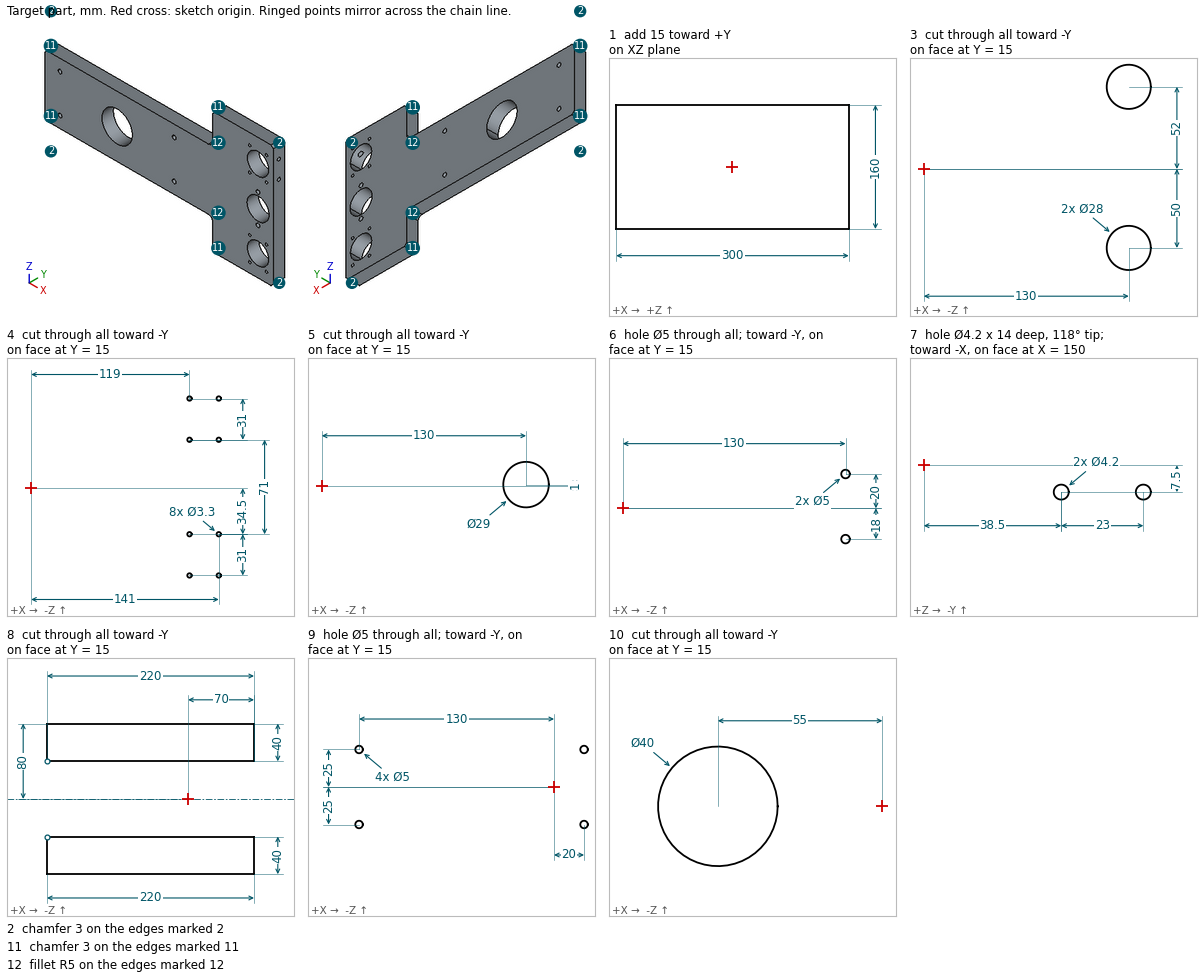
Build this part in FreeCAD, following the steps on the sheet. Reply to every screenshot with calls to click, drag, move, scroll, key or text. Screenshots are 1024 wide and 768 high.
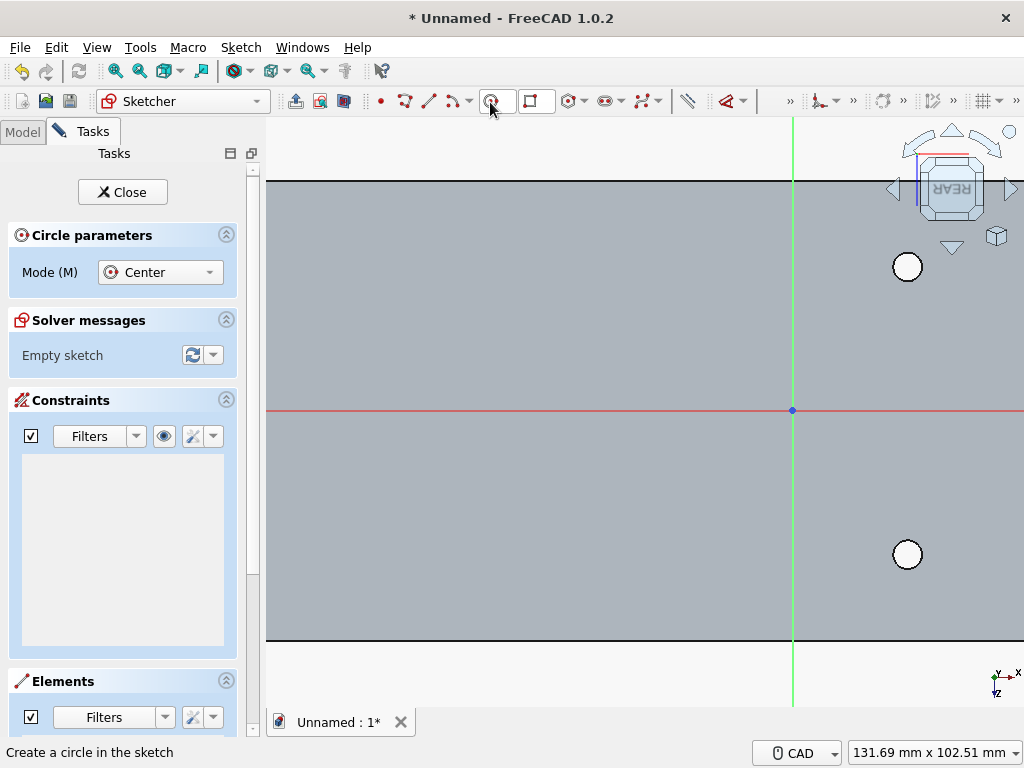
click(476, 411)
move(557, 329)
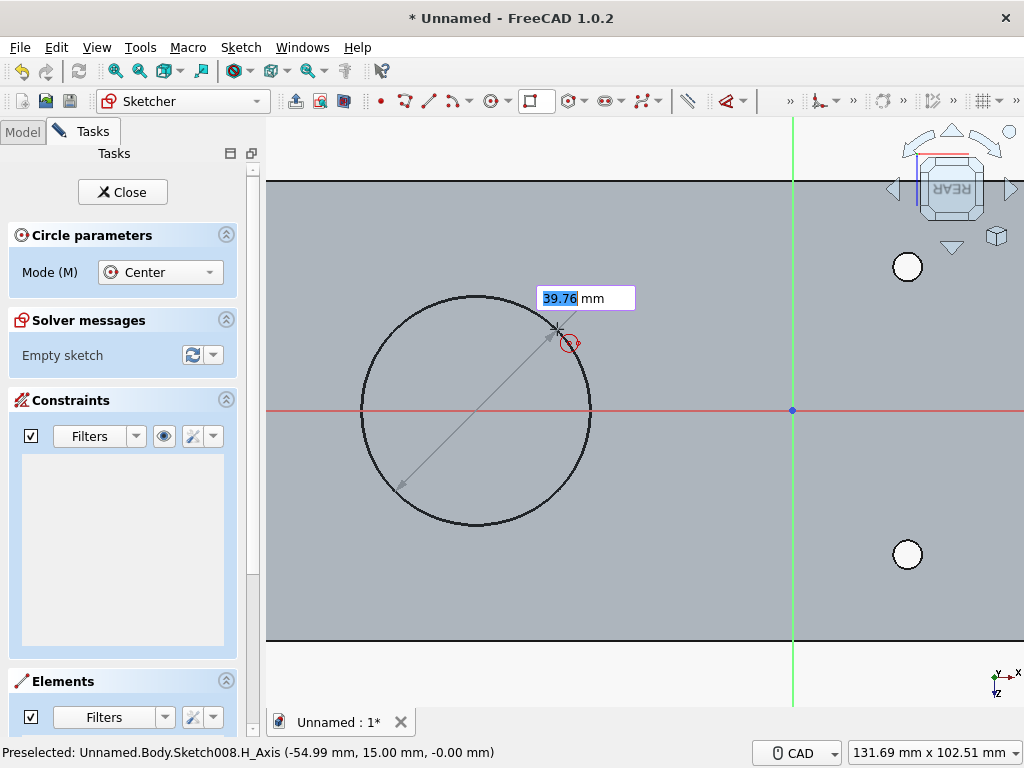
text(40)
key(Return)
key(Escape)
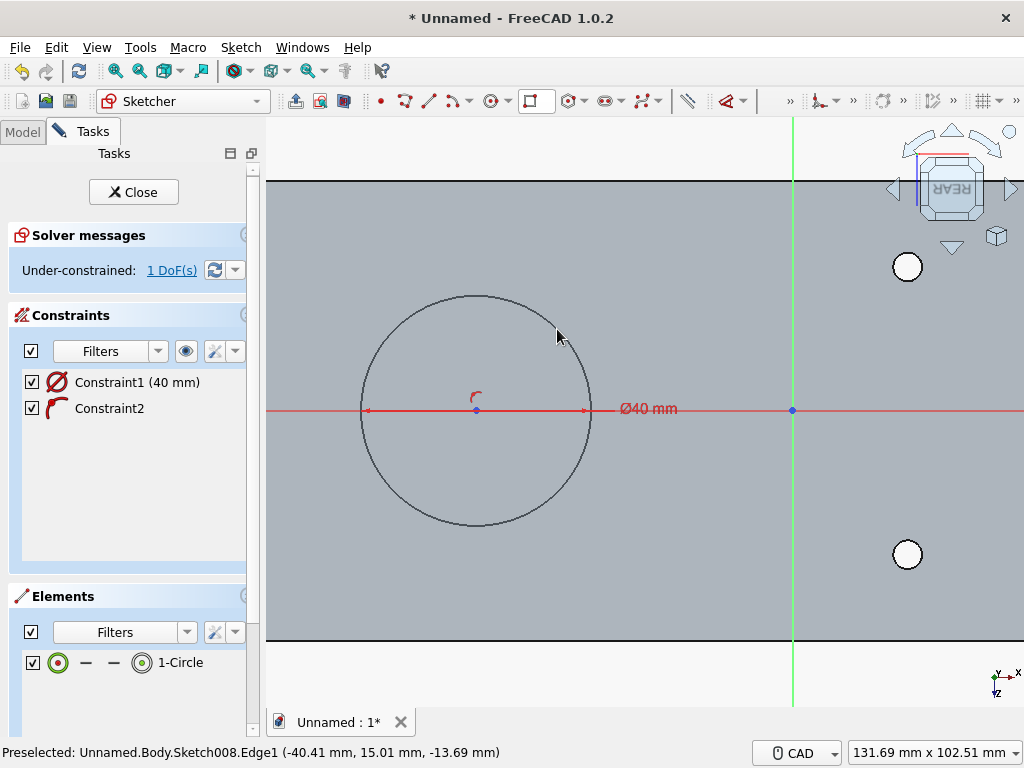
click(726, 102)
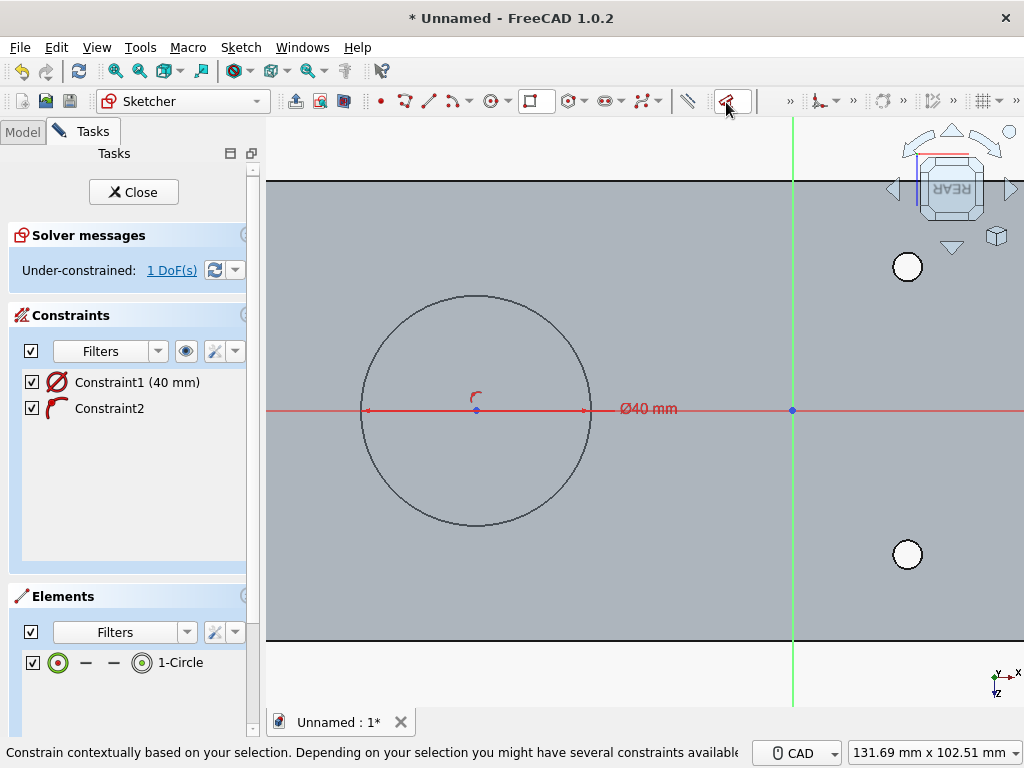
click(476, 411)
click(634, 445)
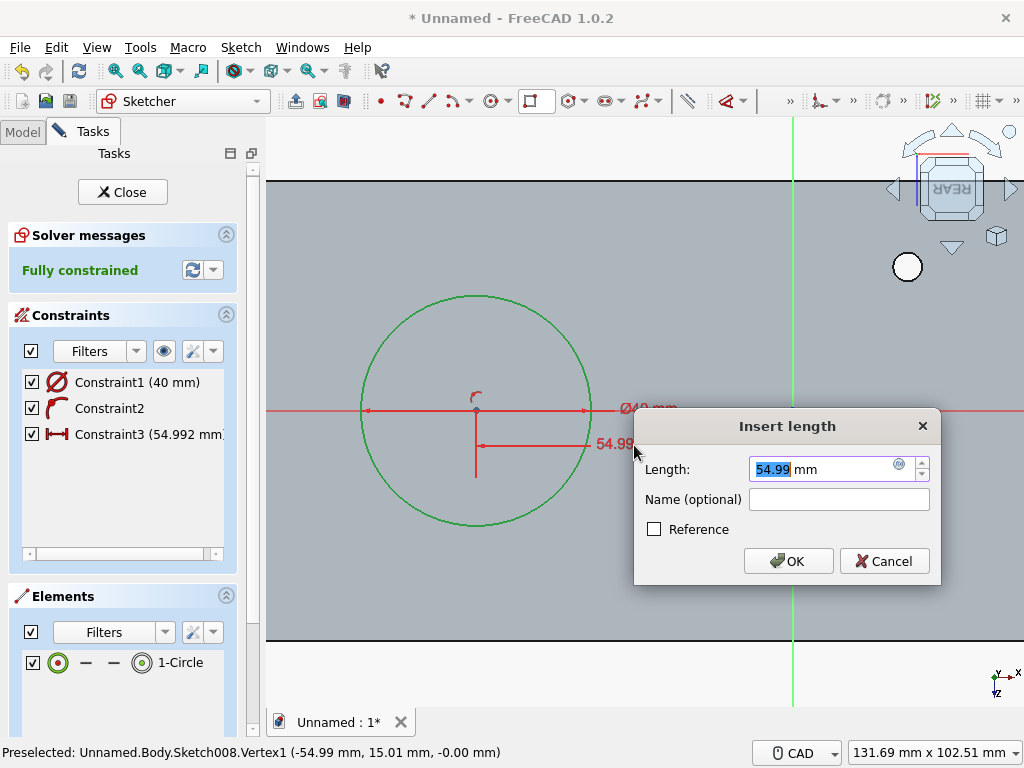
text(55)
key(Return)
key(Escape)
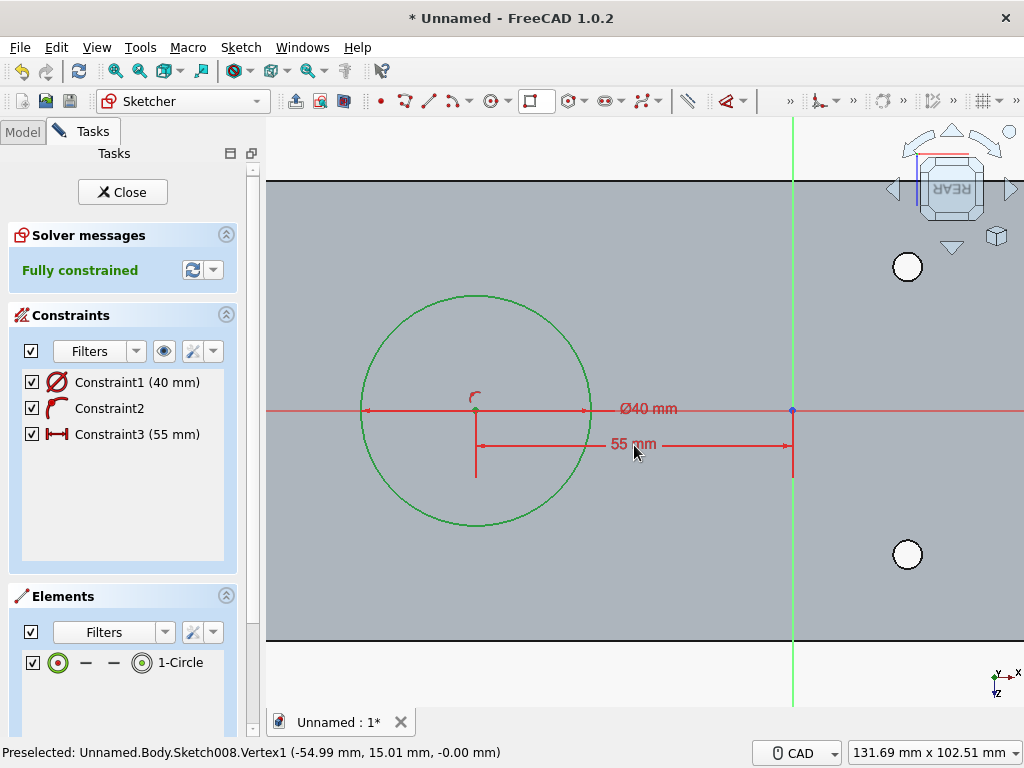
click(123, 192)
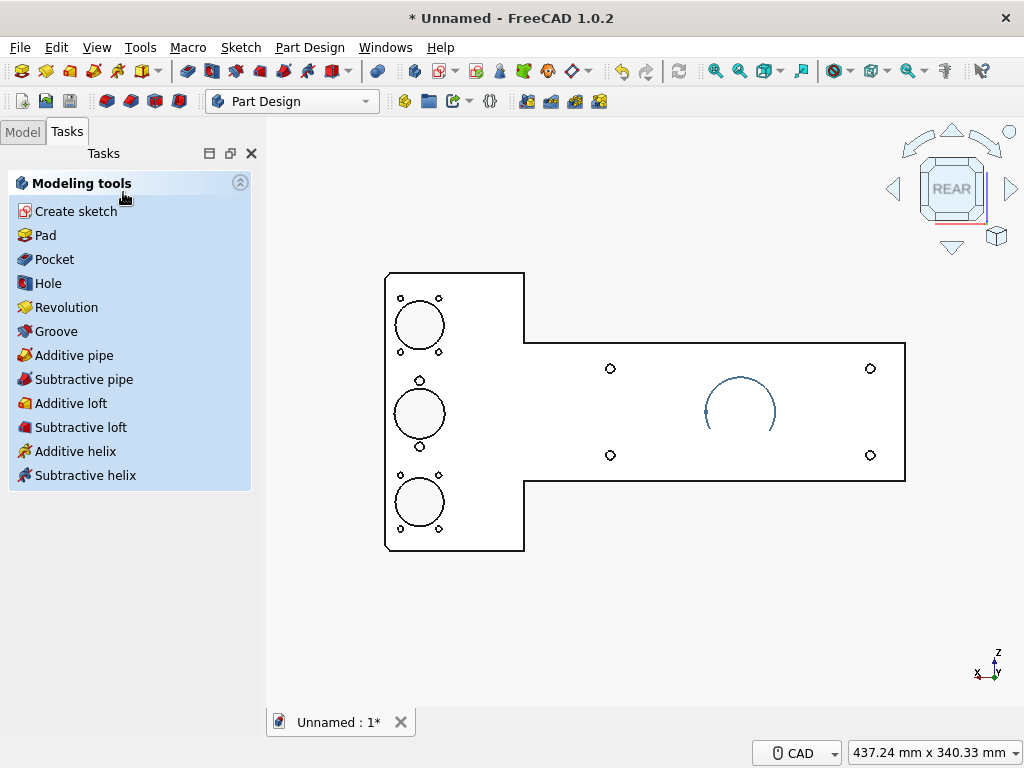
click(188, 72)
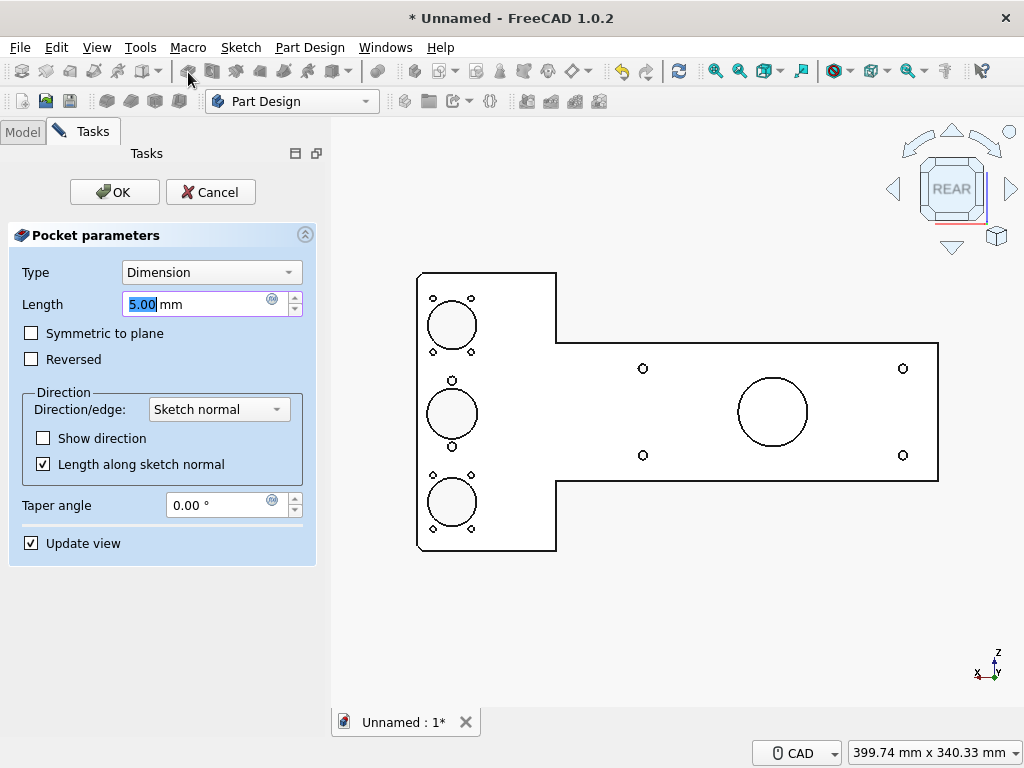
click(212, 272)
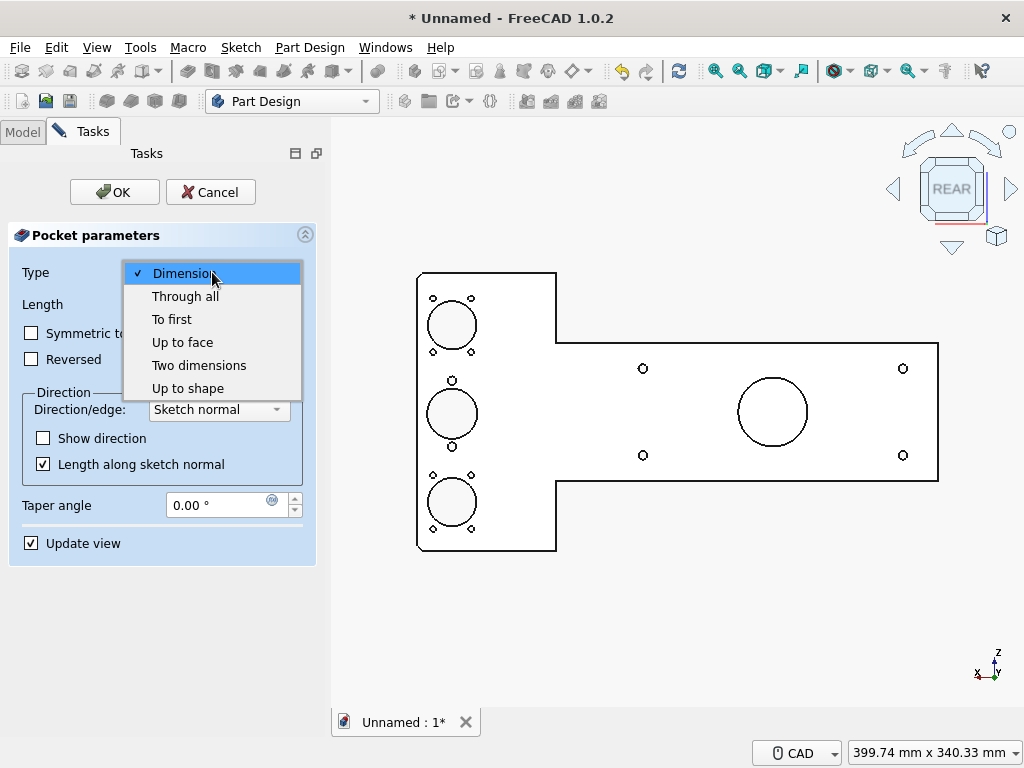
click(212, 296)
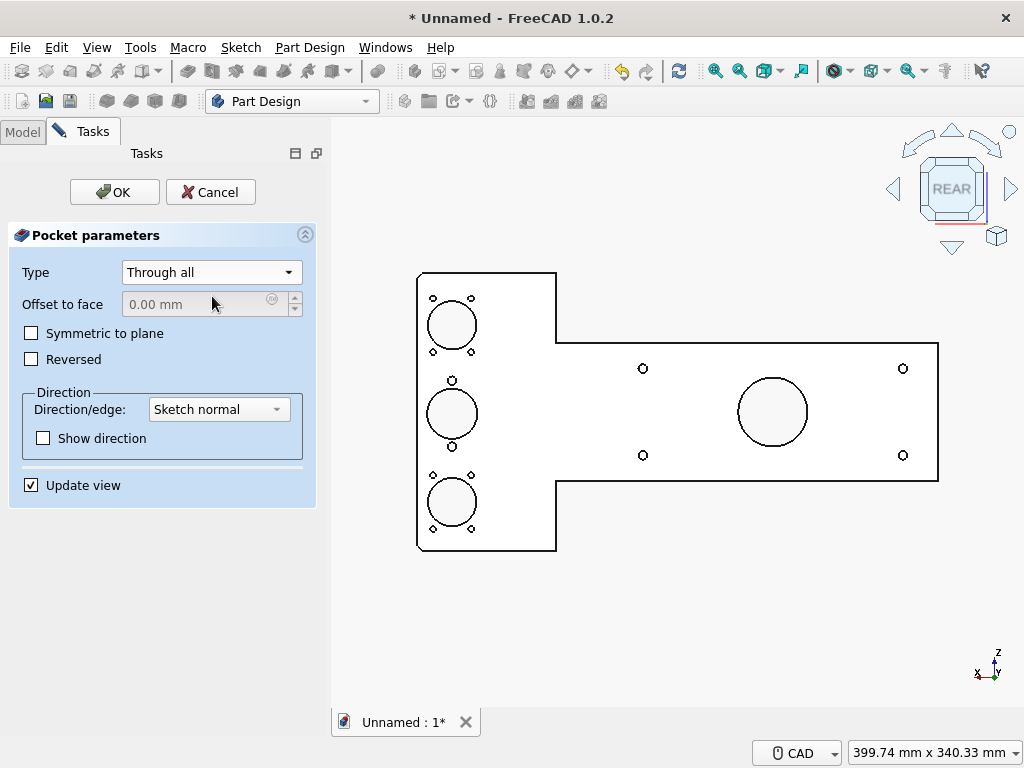
click(115, 192)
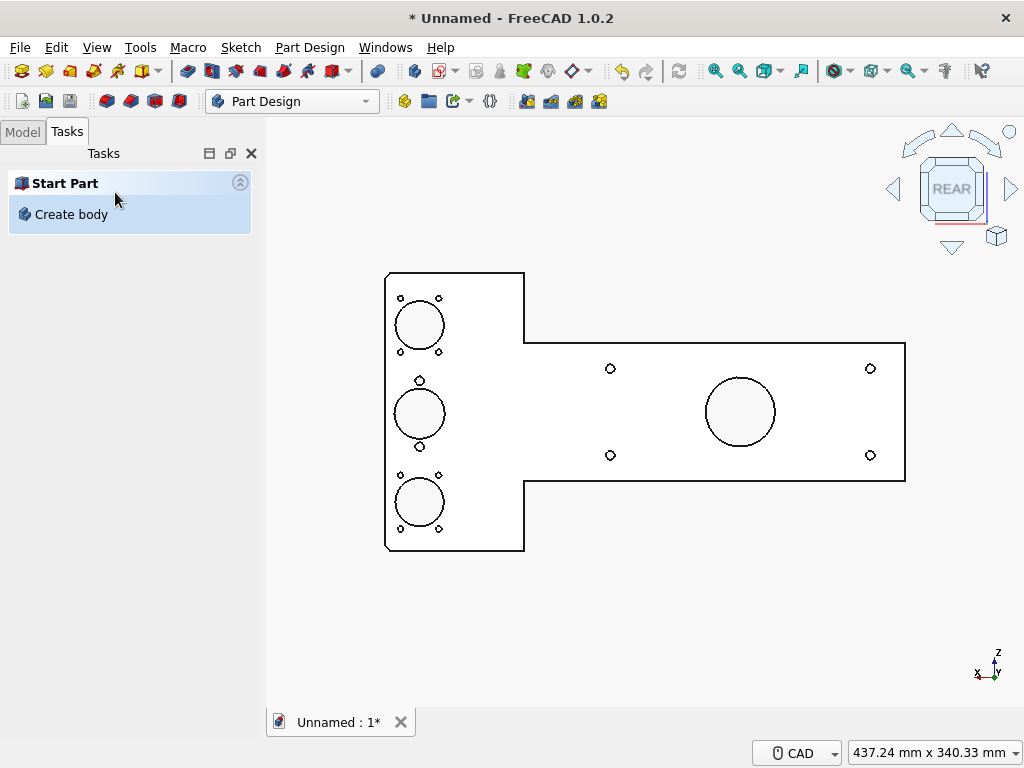
key(0)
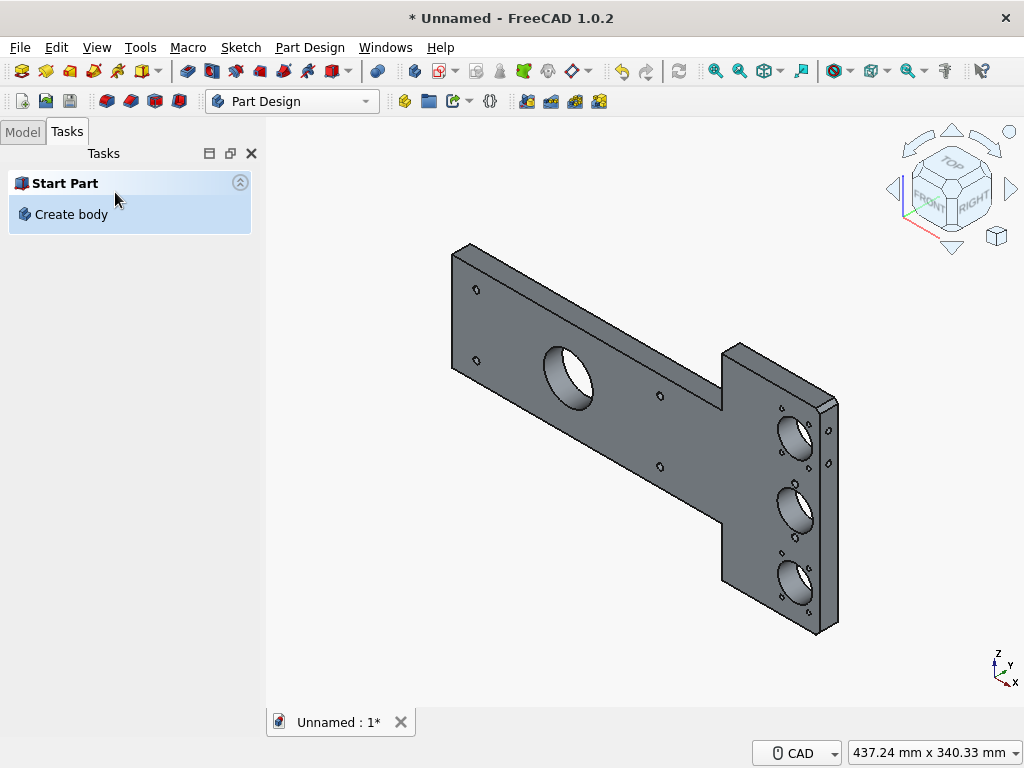
key(2)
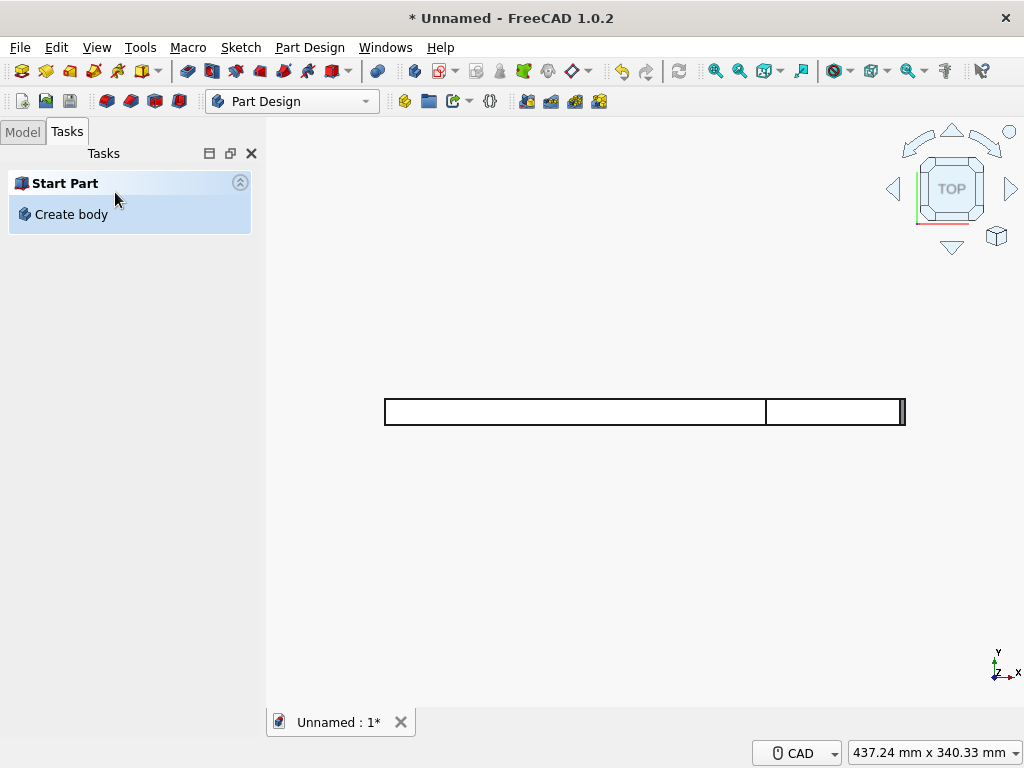
click(385, 411)